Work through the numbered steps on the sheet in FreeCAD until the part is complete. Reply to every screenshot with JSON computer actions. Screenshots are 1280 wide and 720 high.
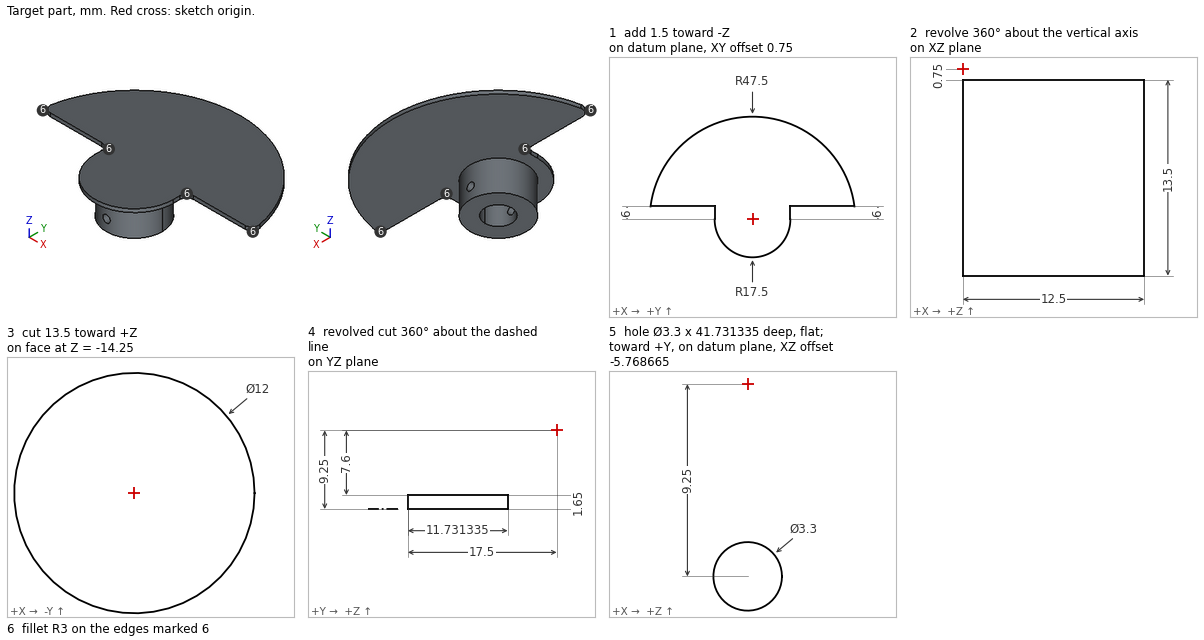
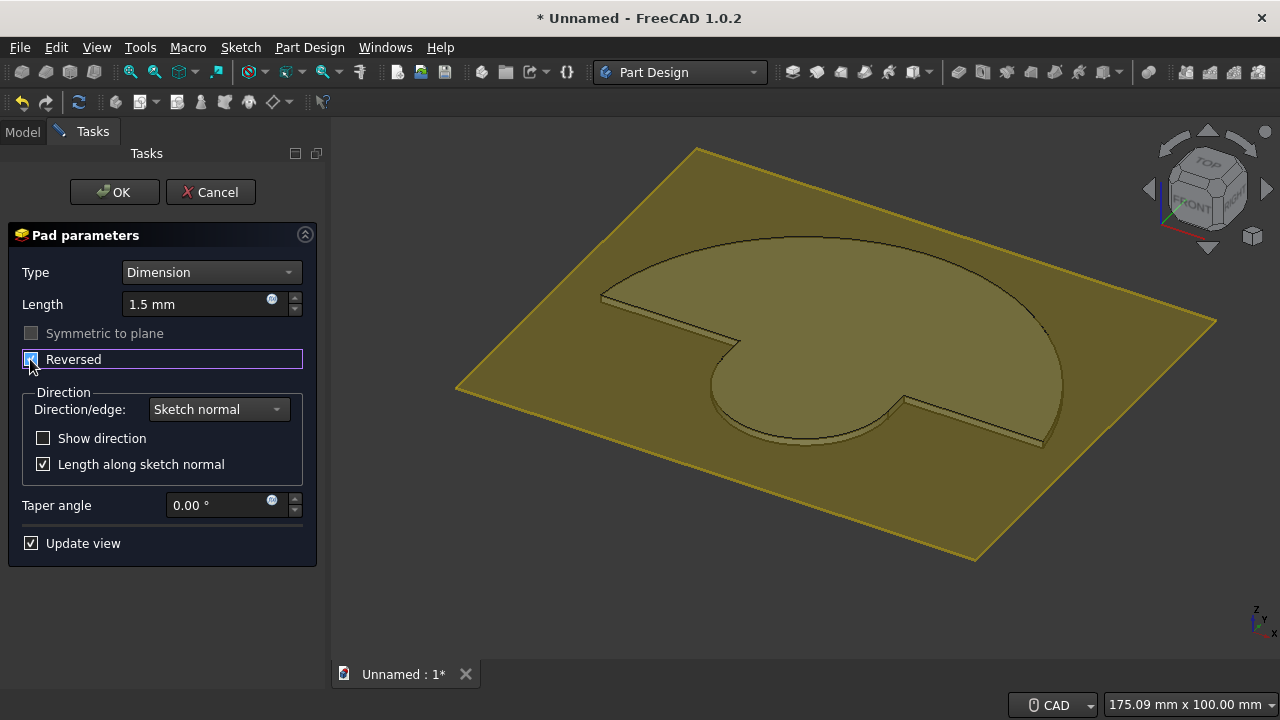
{"action": "left_click", "coordinate": [115, 192]}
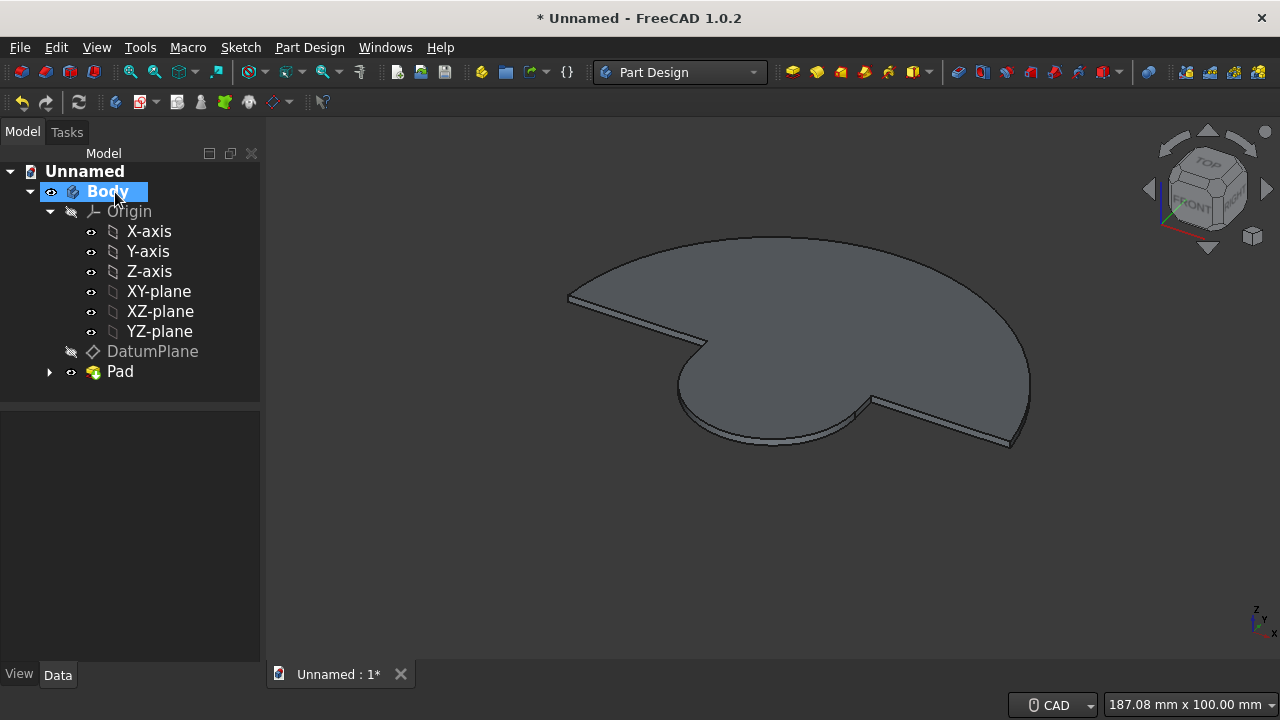
{"action": "left_click", "coordinate": [140, 102]}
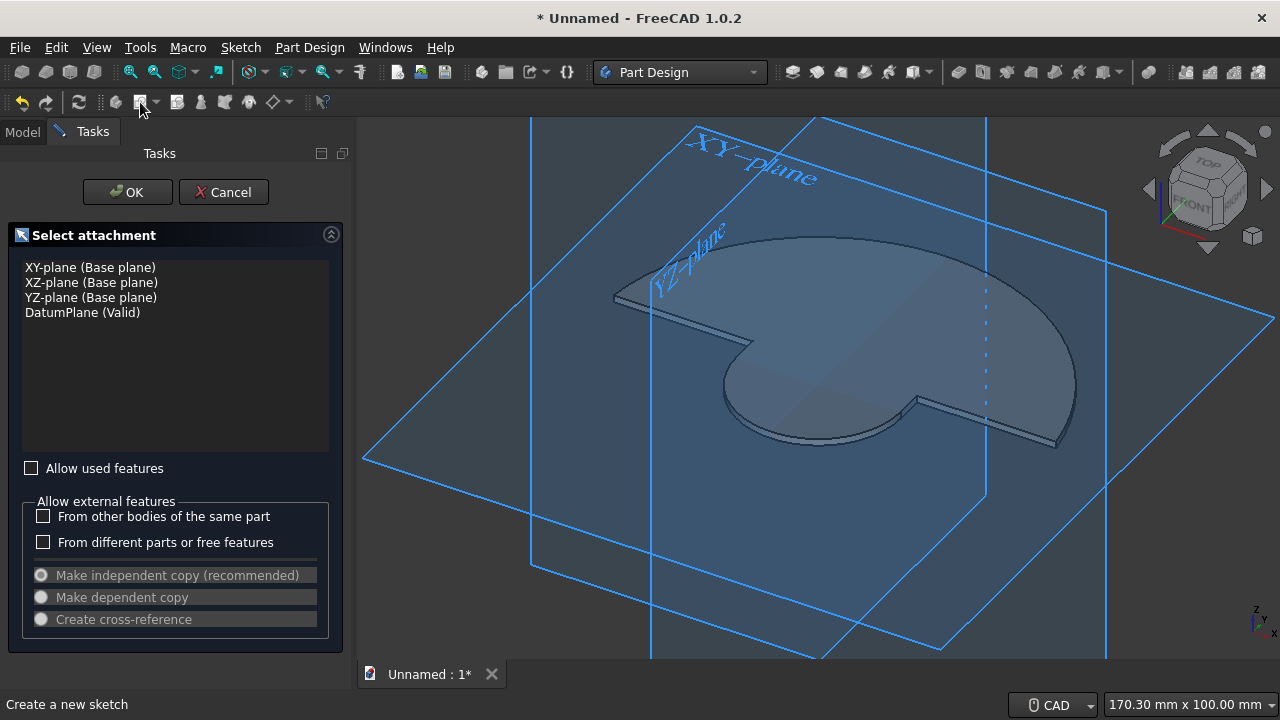
{"action": "left_click", "coordinate": [82, 282]}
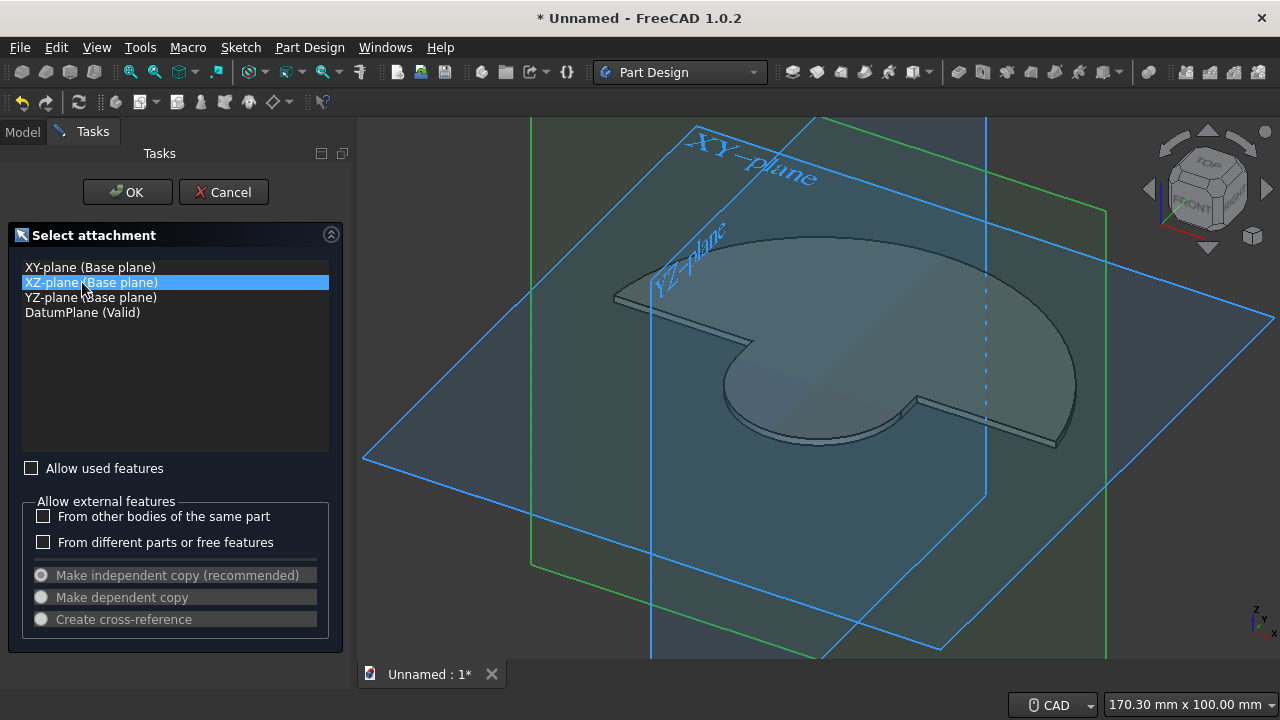
{"action": "left_click", "coordinate": [128, 192]}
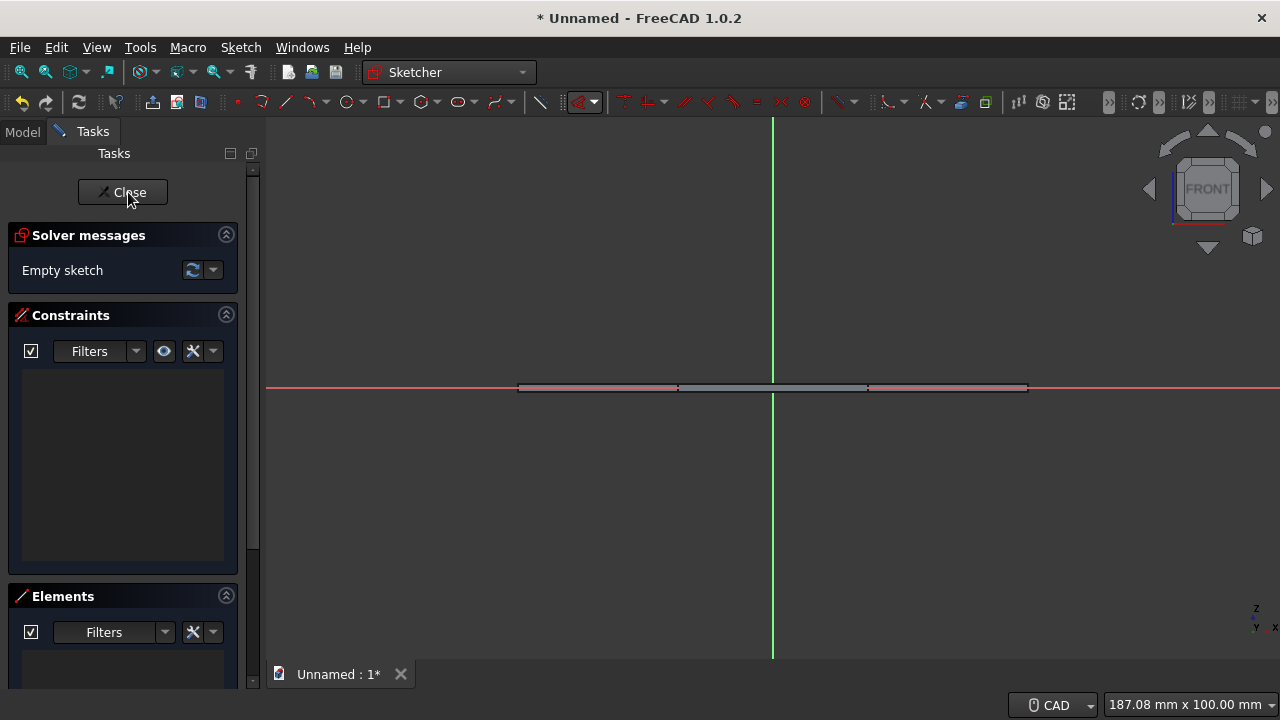
{"action": "left_click", "coordinate": [202, 102]}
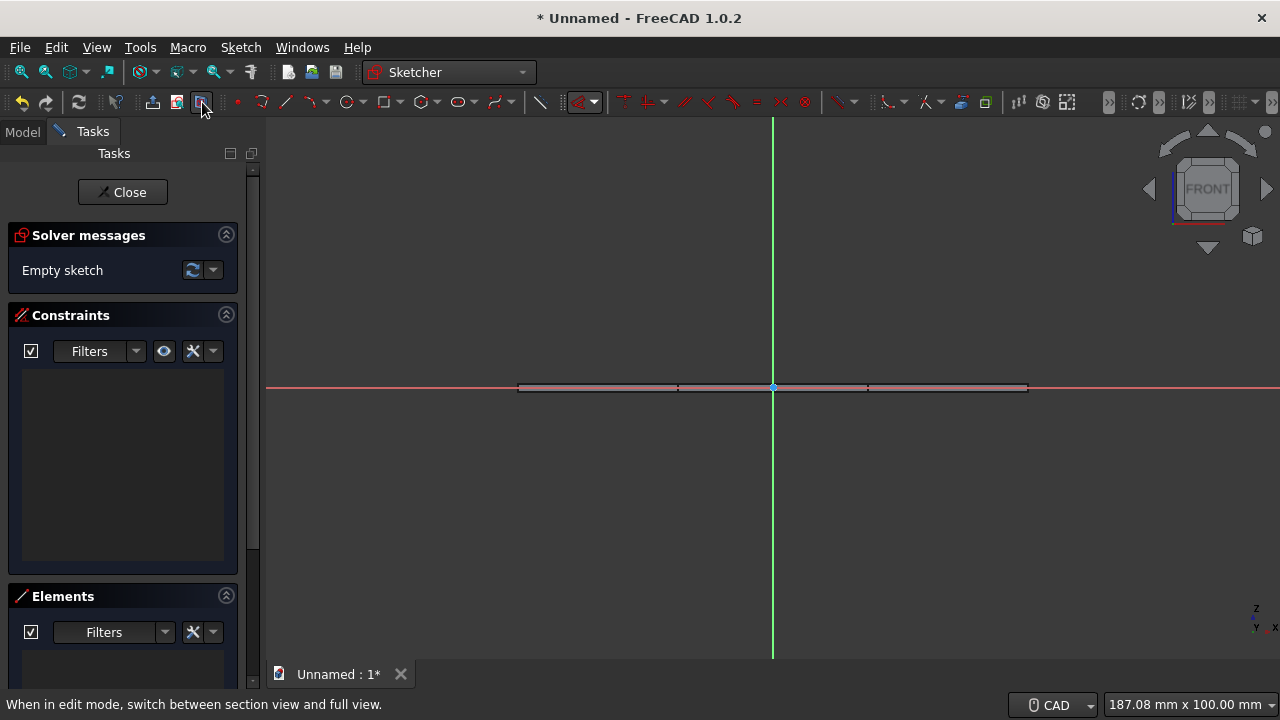
{"action": "scroll", "coordinate": [840, 439], "scroll_direction": "up", "scroll_amount": 7}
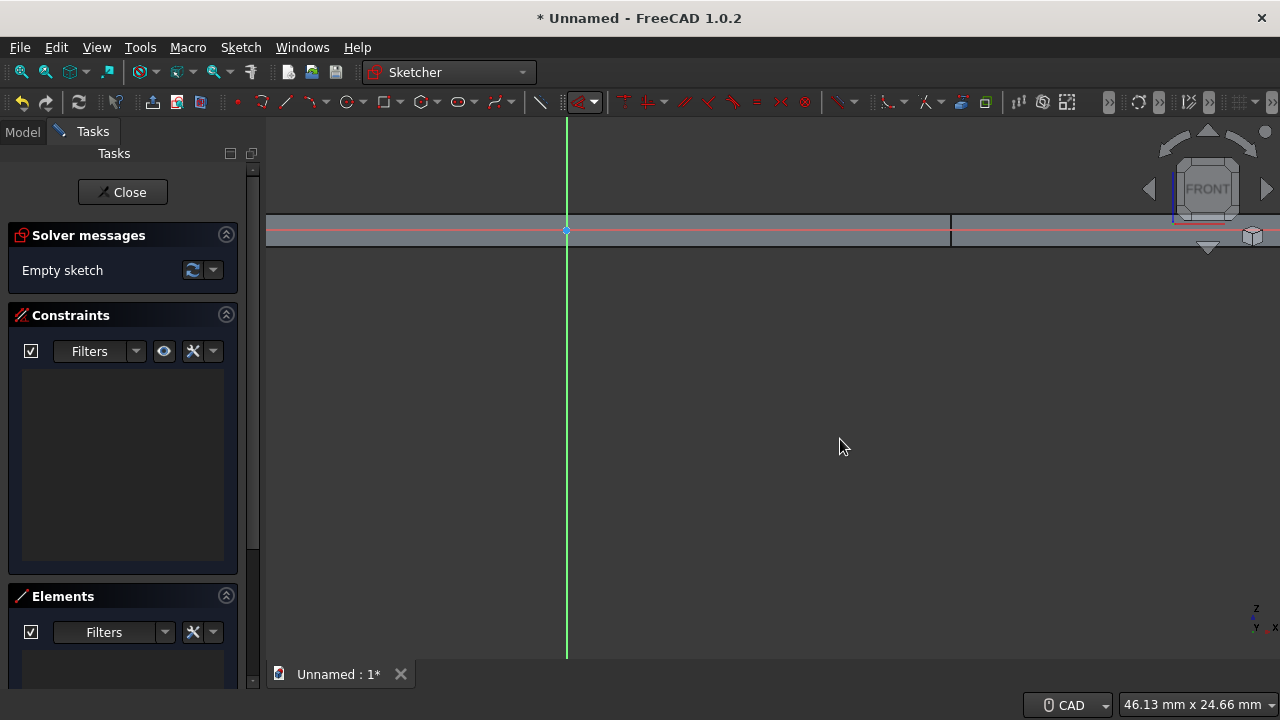
{"action": "key", "text": "g r"}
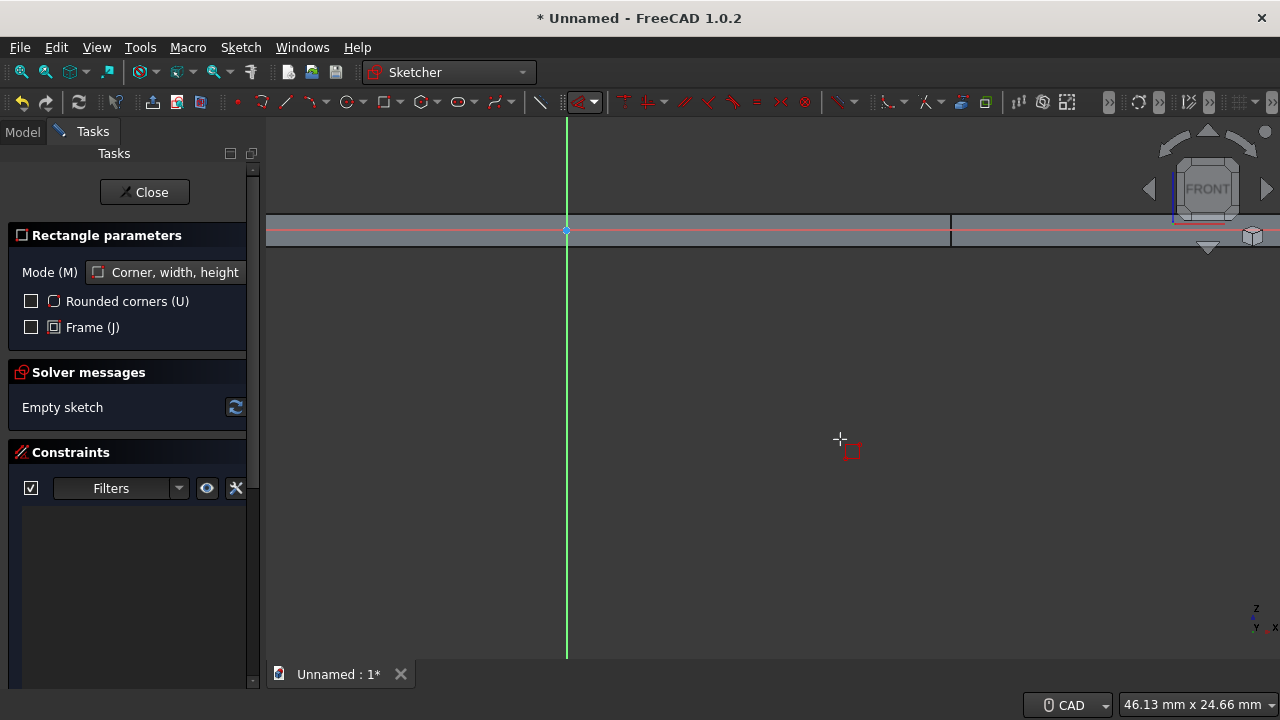
{"action": "left_click", "coordinate": [567, 247]}
{"action": "mouse_move", "coordinate": [841, 544]}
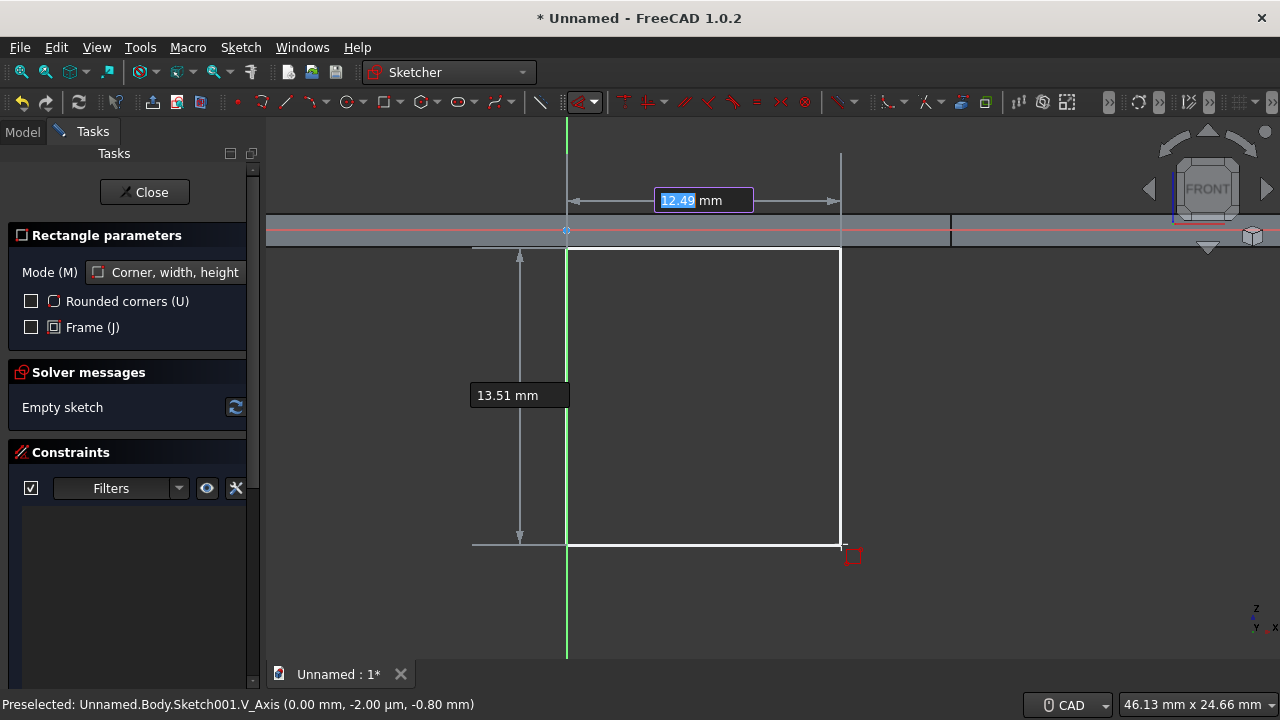
{"action": "type", "text": "12.5"}
{"action": "key", "text": "Tab"}
{"action": "type", "text": "13.5"}
{"action": "key", "text": "Return"}
{"action": "key", "text": "Escape"}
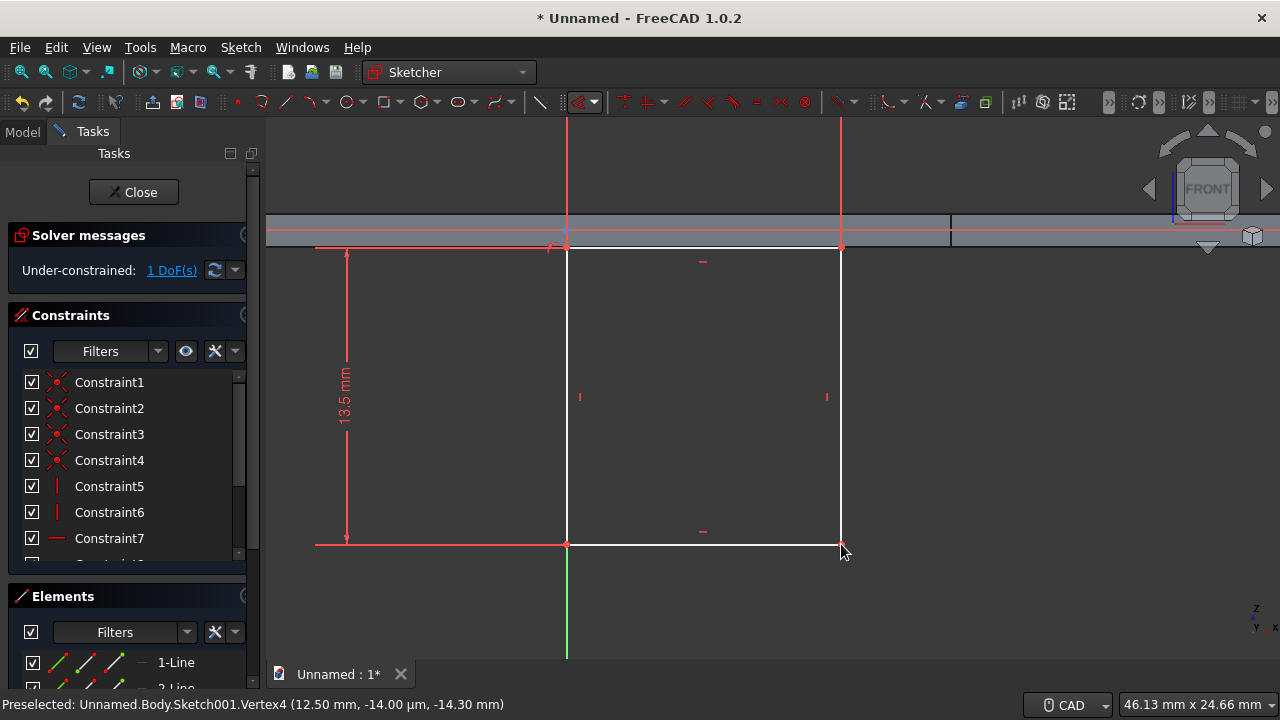
{"action": "left_click", "coordinate": [578, 102]}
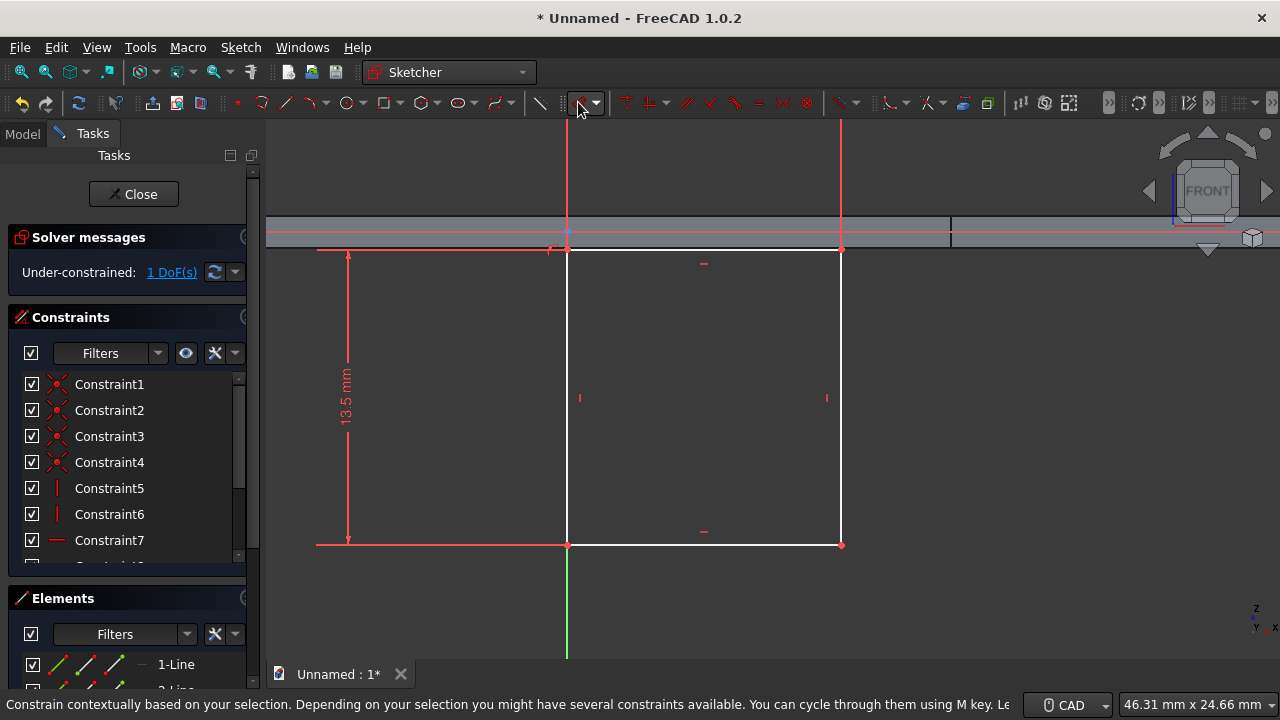
{"action": "scroll", "coordinate": [567, 250], "scroll_direction": "up", "scroll_amount": 5}